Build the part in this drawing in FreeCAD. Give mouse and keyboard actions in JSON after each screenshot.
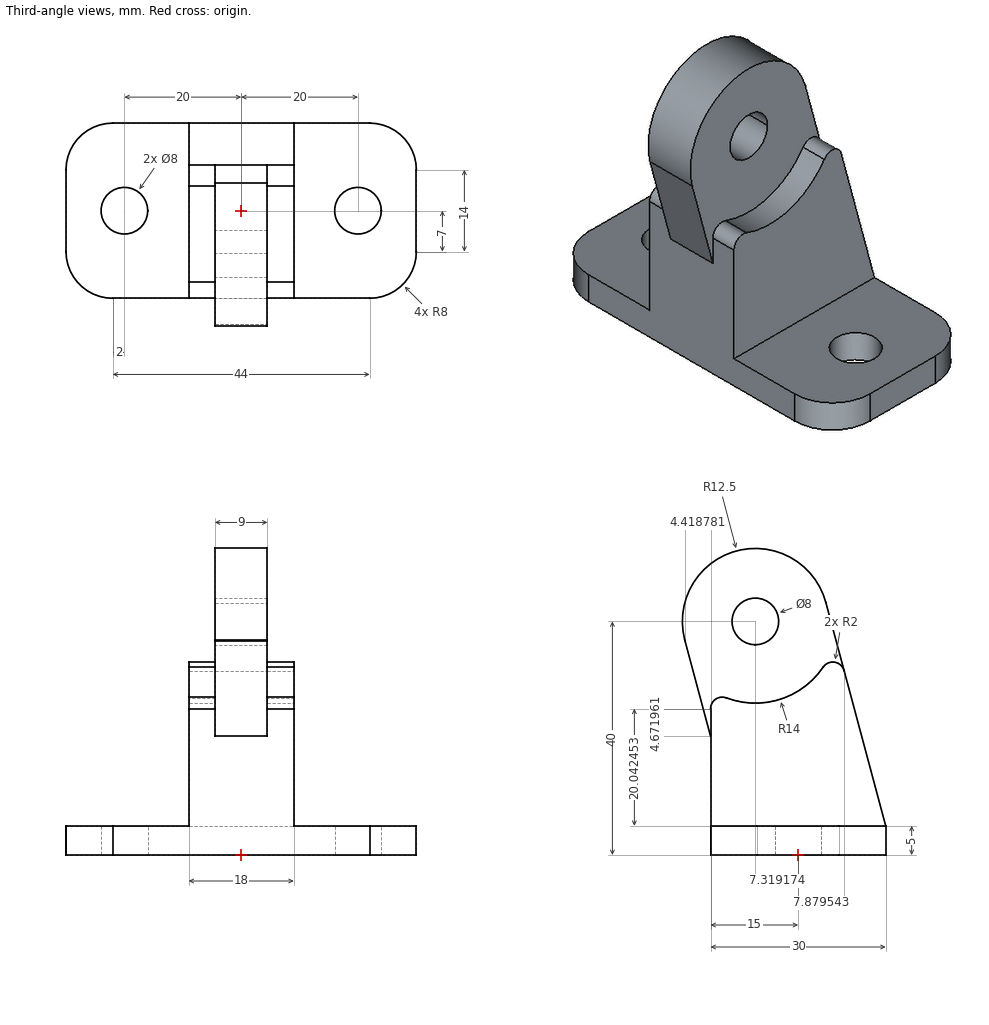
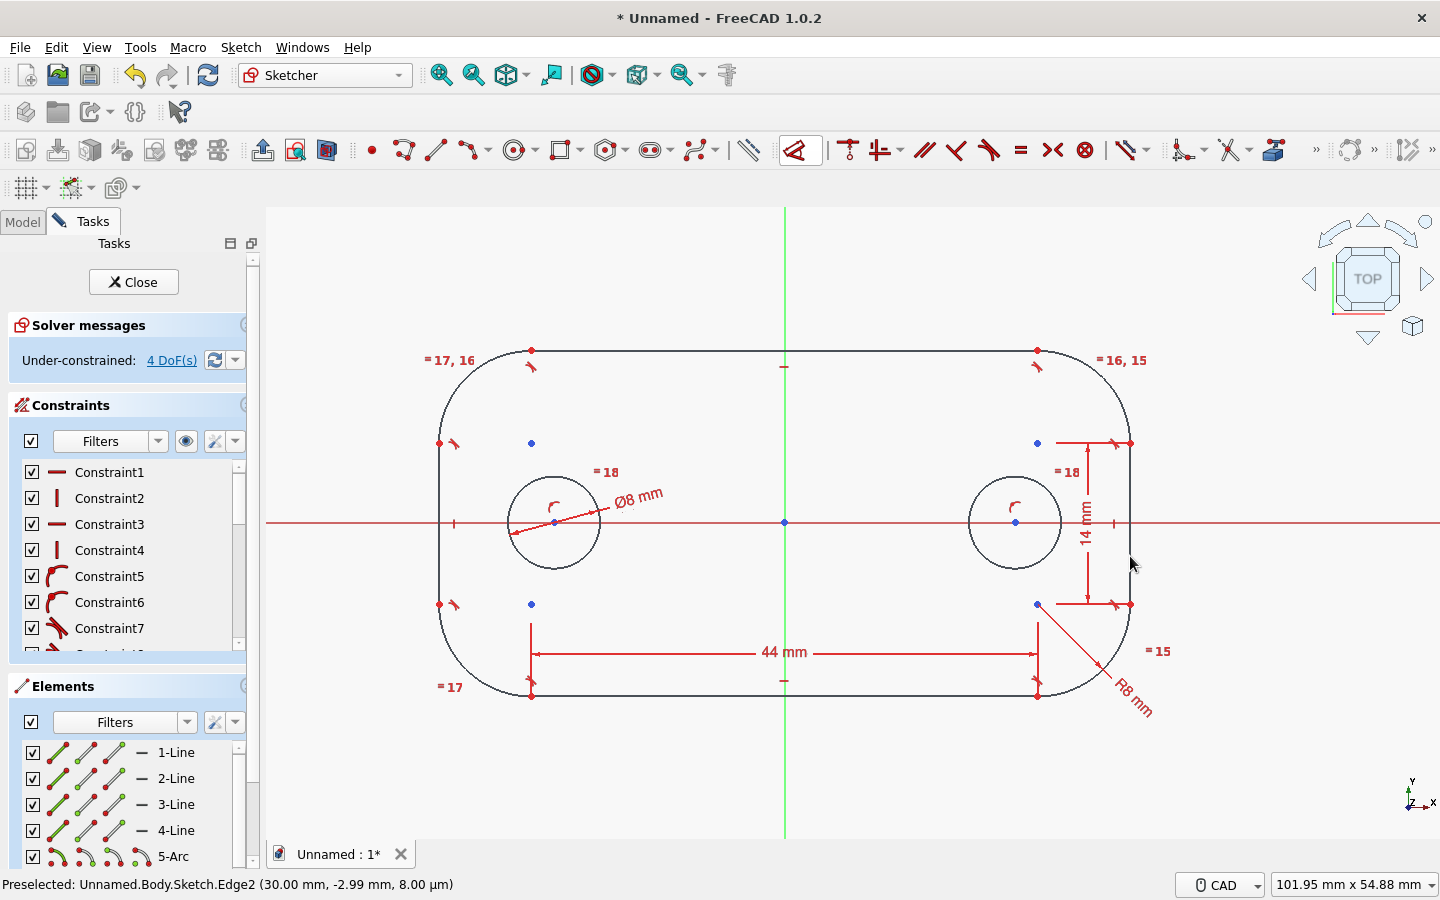
{"action": "left_click", "coordinate": [1130, 604]}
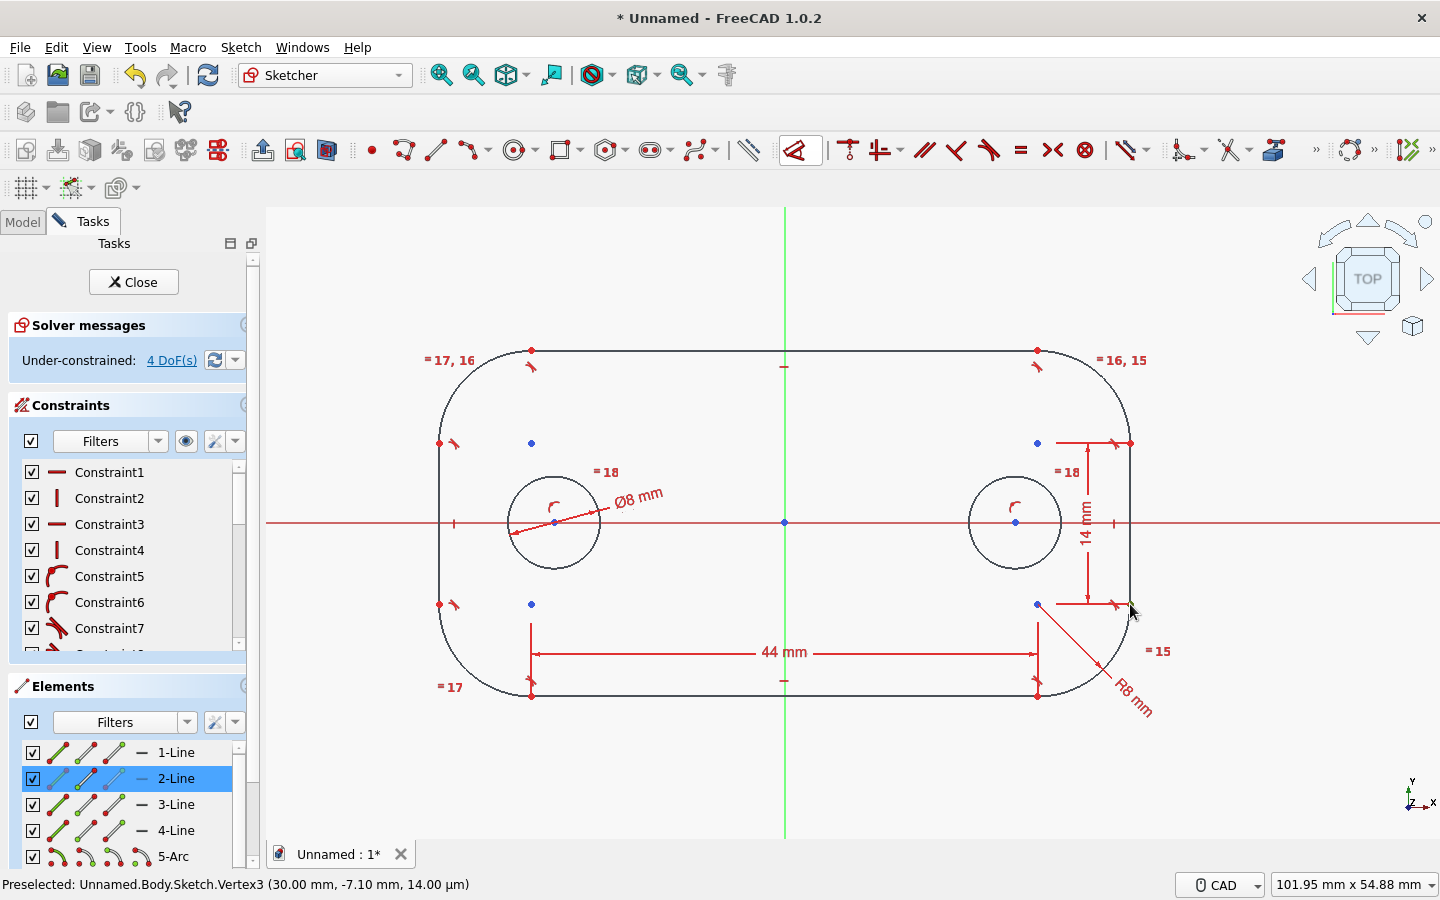
{"action": "key", "text": "i"}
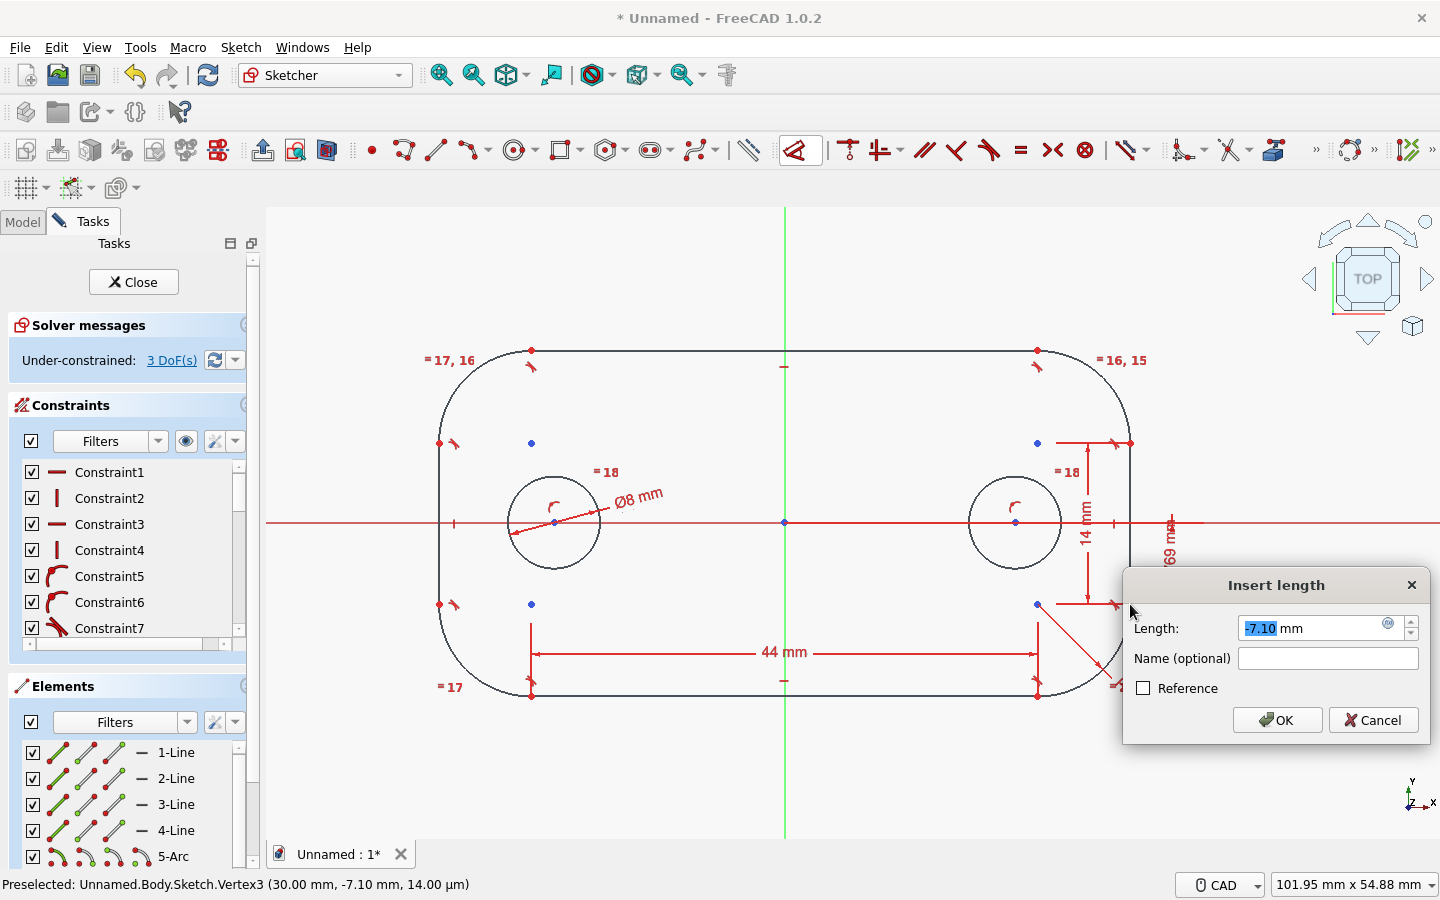
{"action": "type", "text": "-7"}
{"action": "key", "text": "Return"}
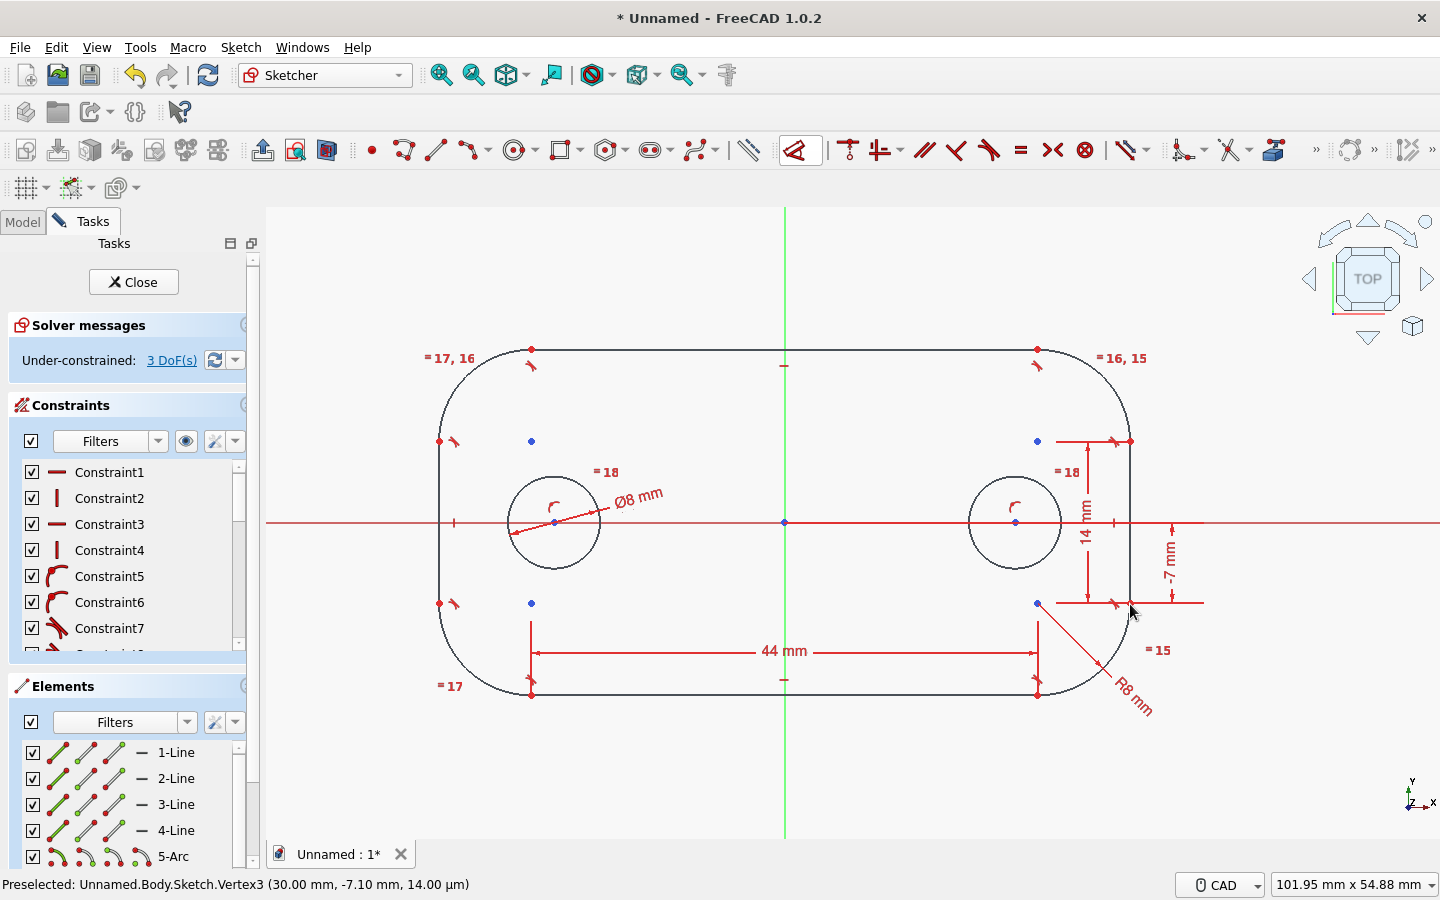
{"action": "left_click", "coordinate": [554, 523]}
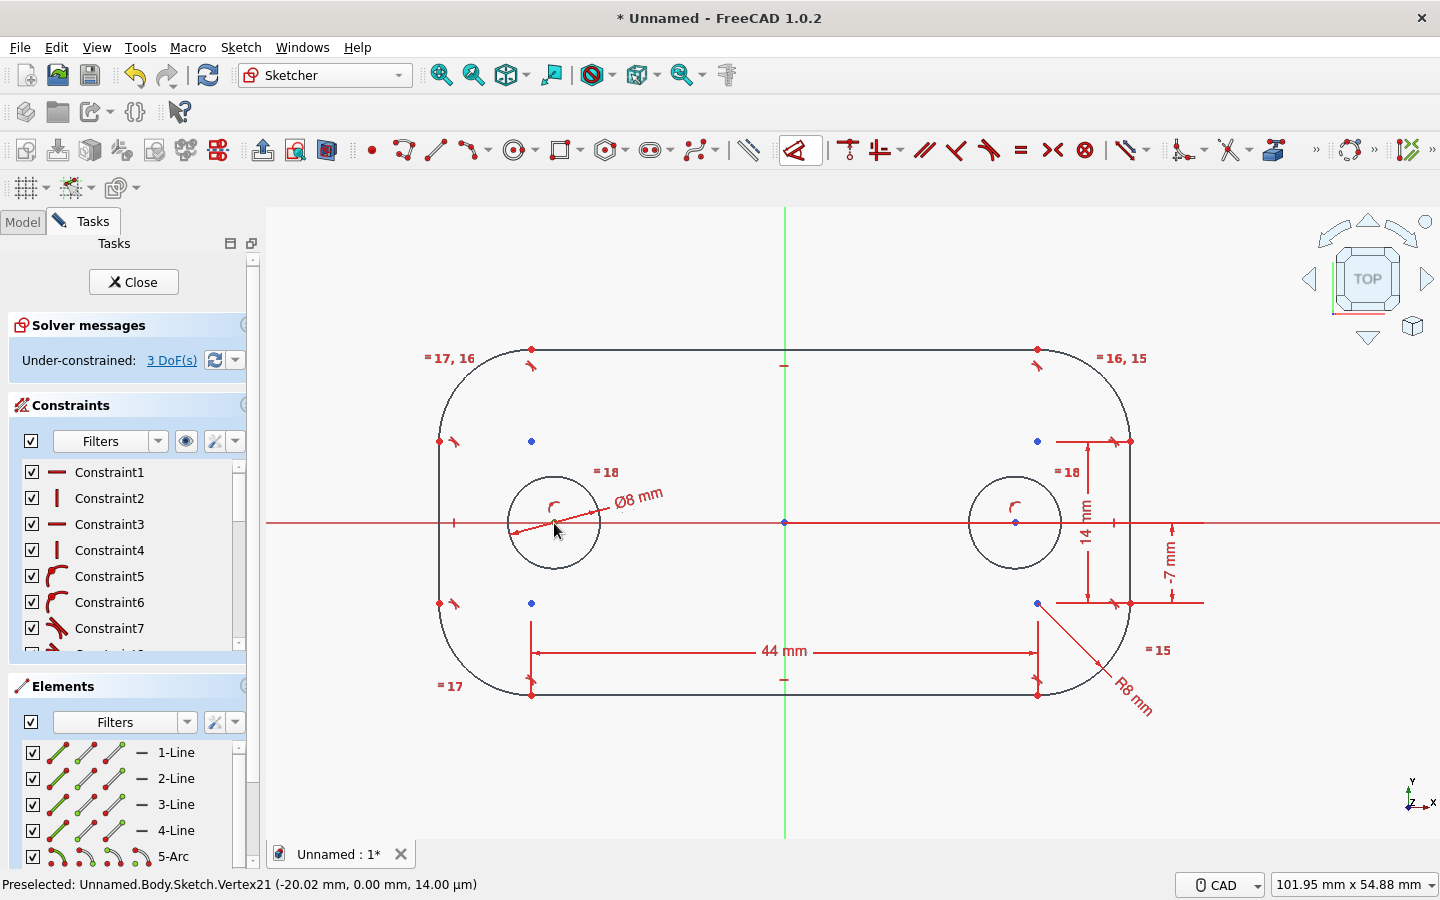
{"action": "key", "text": "l"}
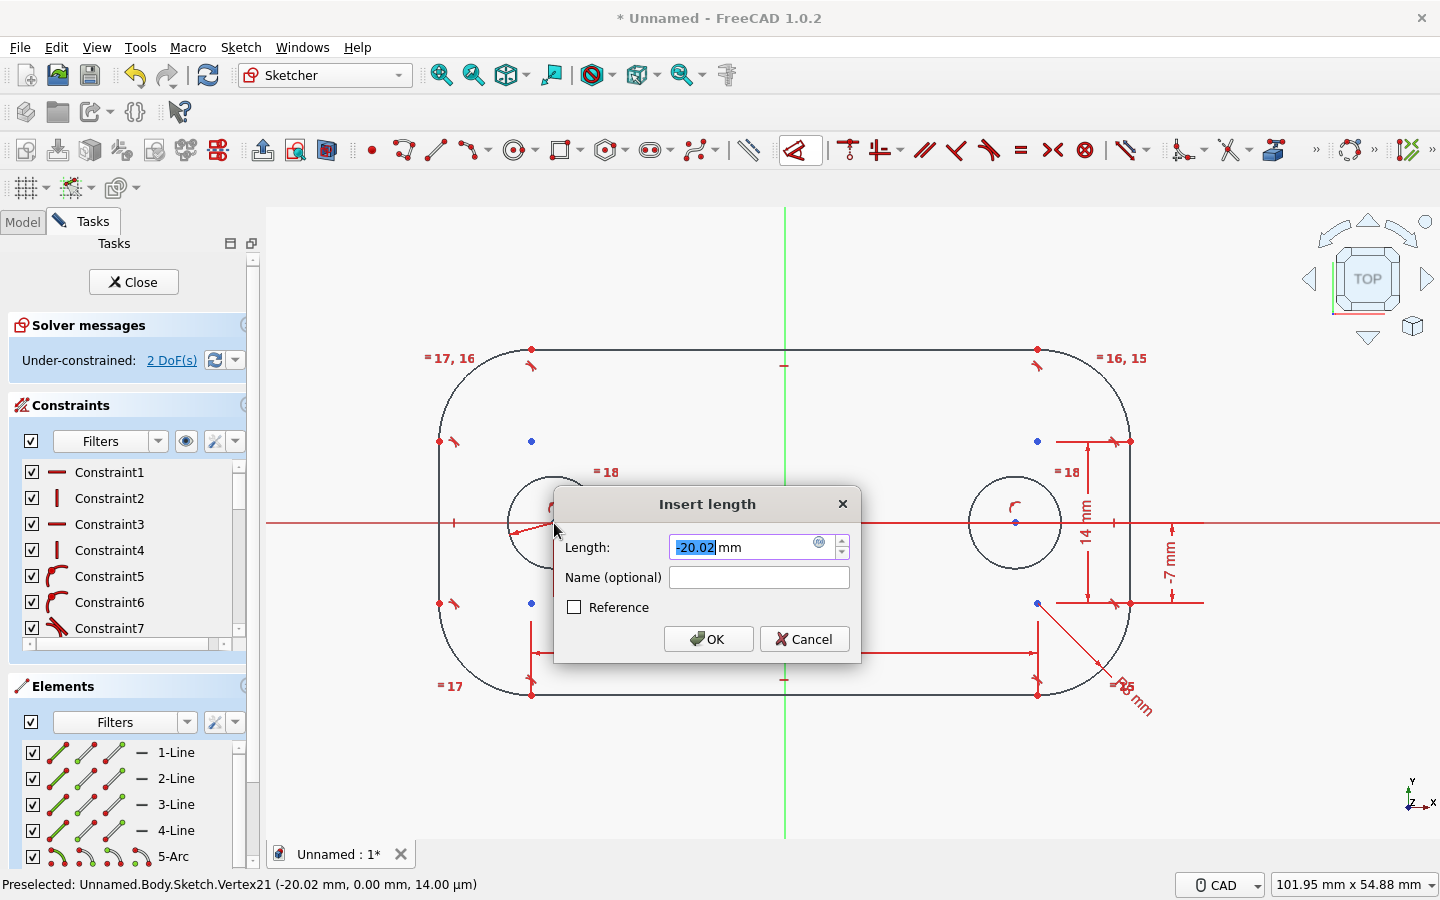
{"action": "type", "text": "-20"}
{"action": "key", "text": "Return"}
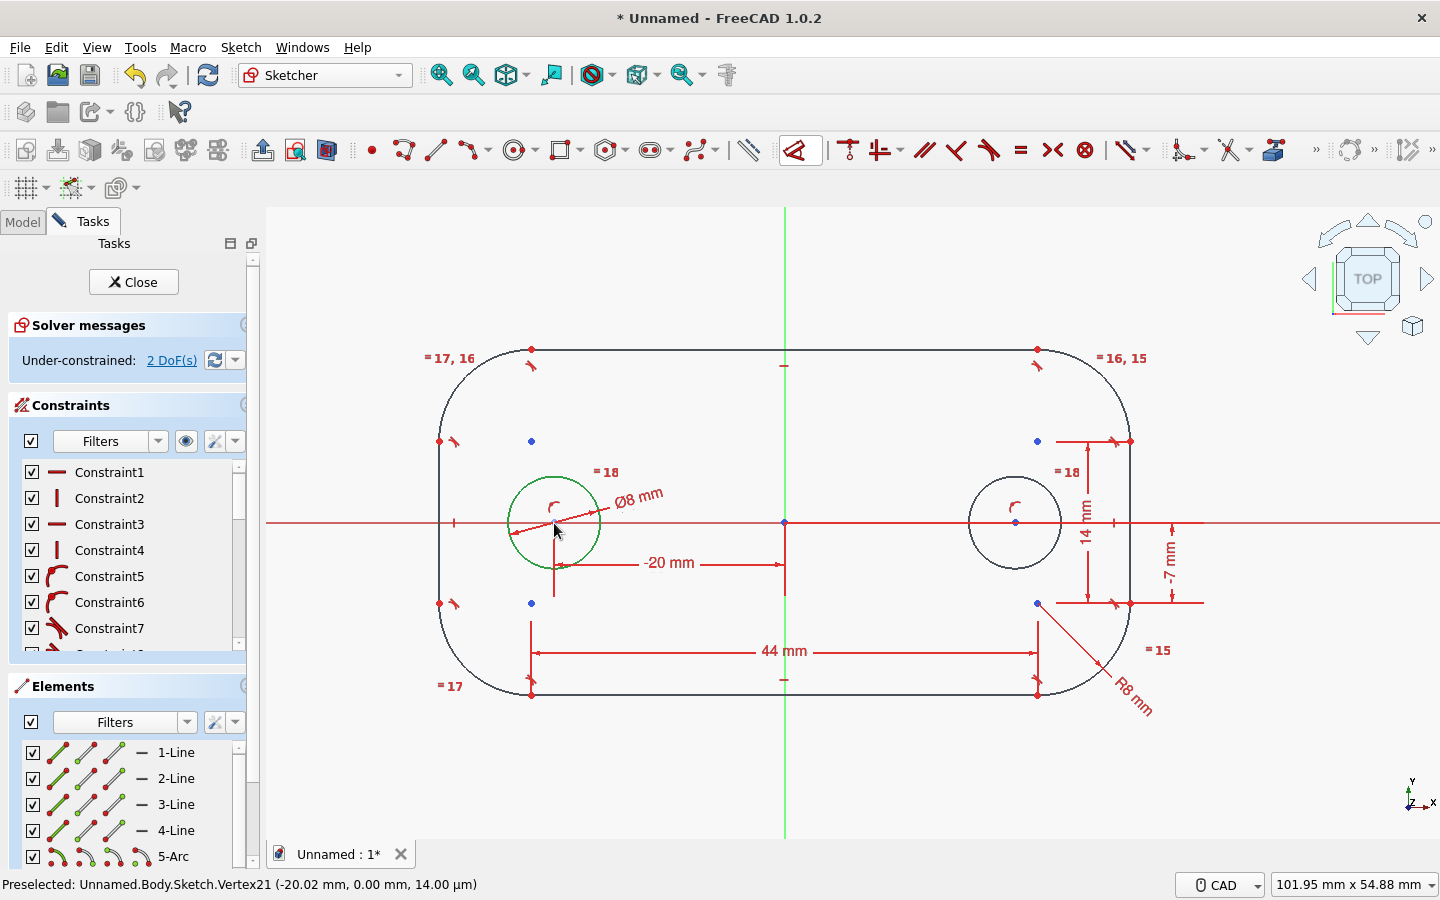
{"action": "left_click", "coordinate": [1015, 523]}